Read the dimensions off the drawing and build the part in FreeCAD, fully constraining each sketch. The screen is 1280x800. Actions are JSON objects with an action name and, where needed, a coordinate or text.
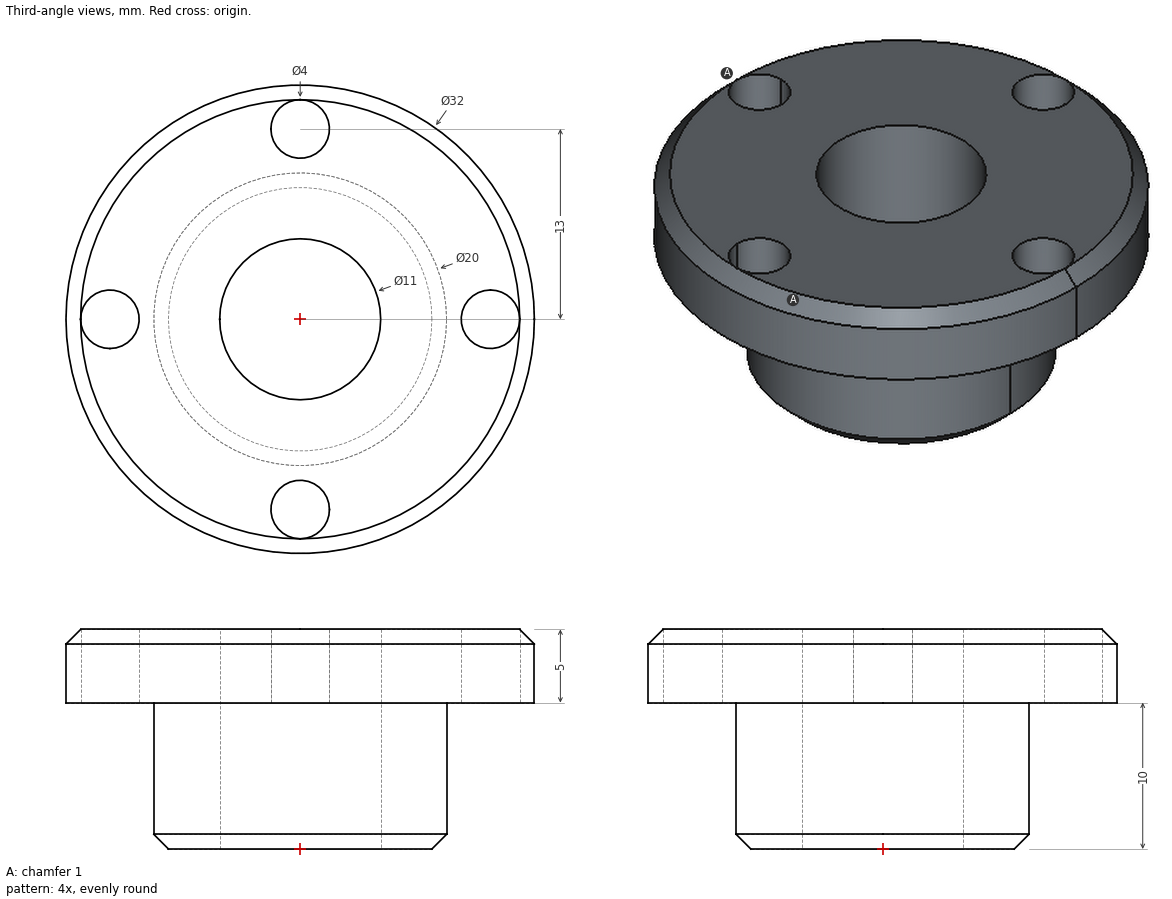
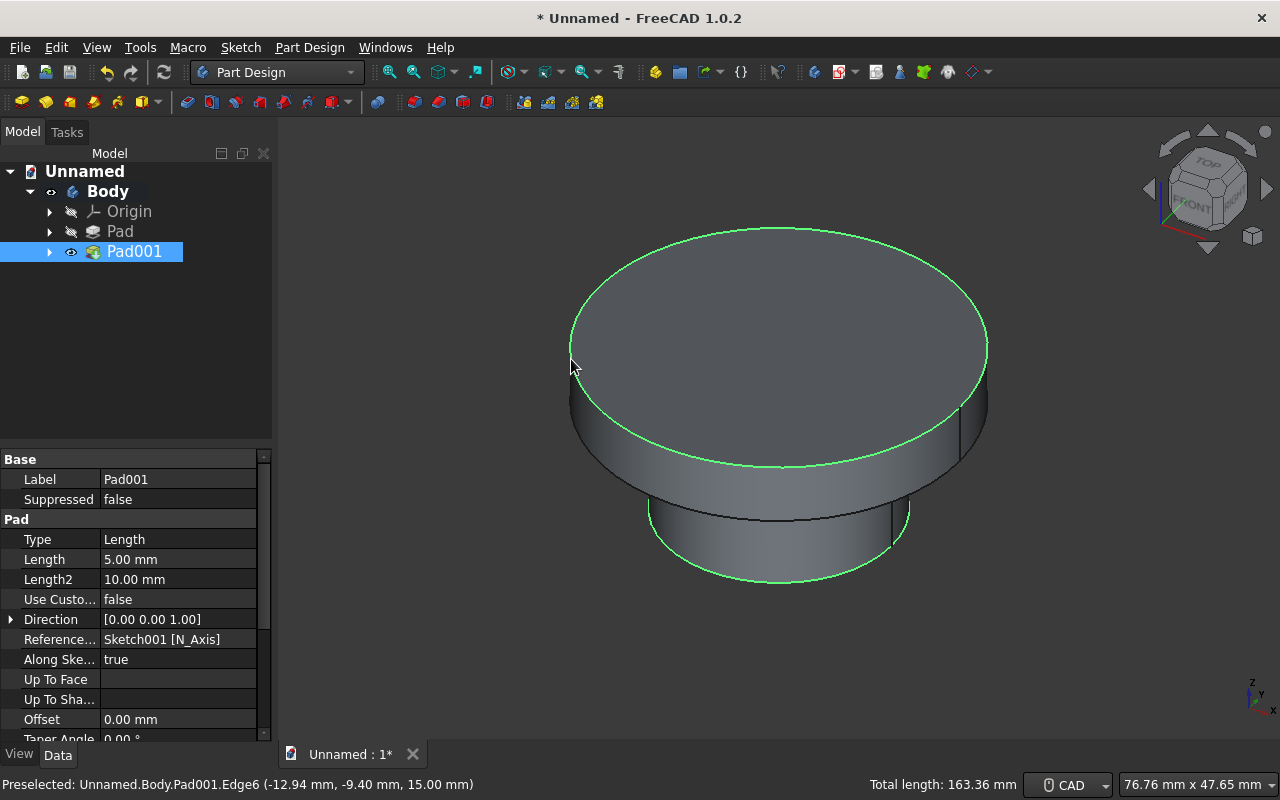
{"action": "left_click", "coordinate": [440, 102]}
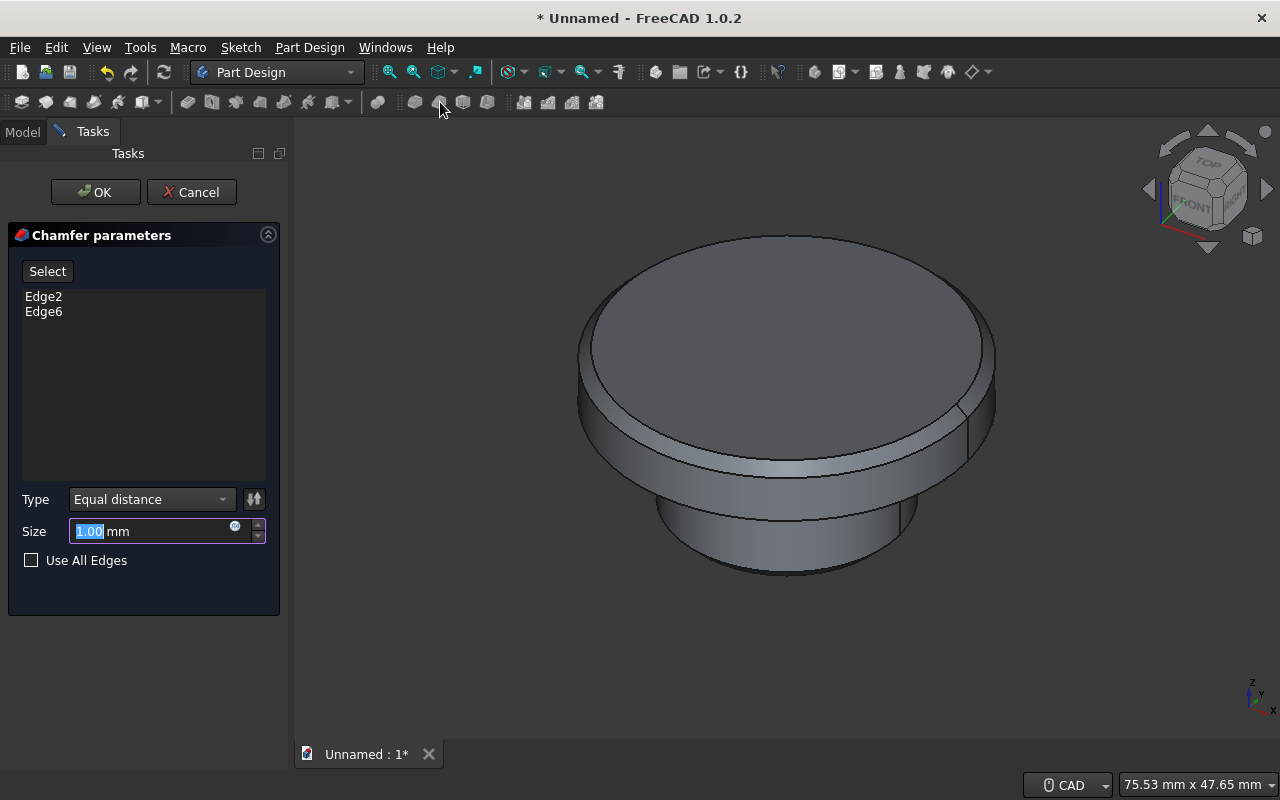
{"action": "type", "text": "1"}
{"action": "key", "text": "Tab"}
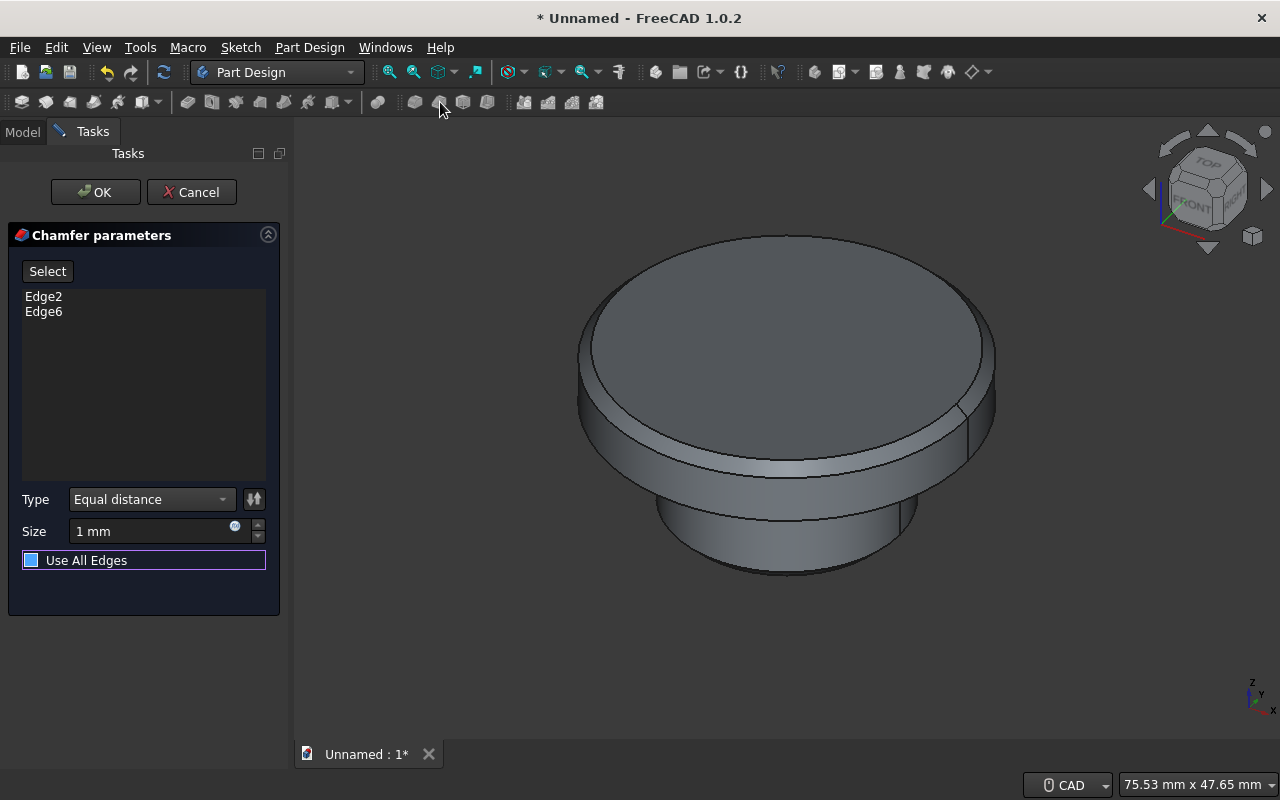
{"action": "left_click", "coordinate": [96, 192]}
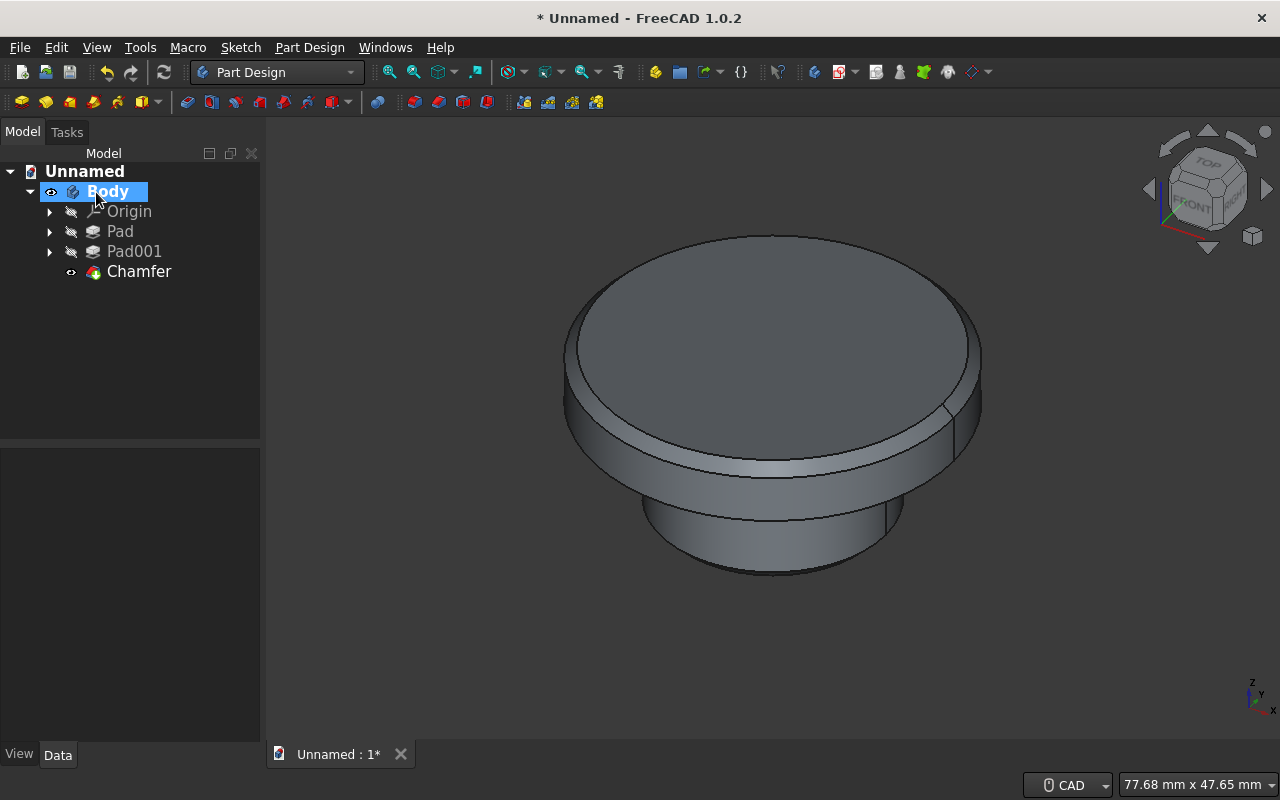
{"action": "key", "text": "5"}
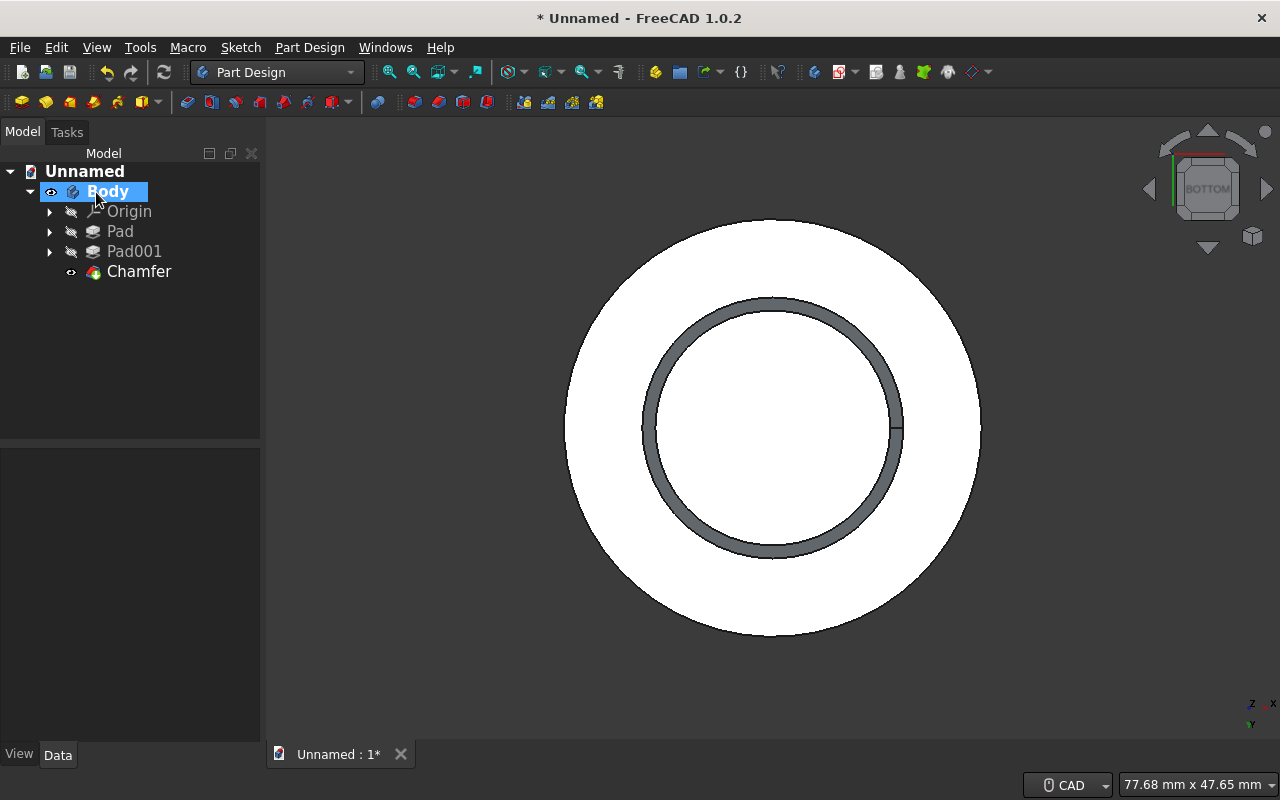
{"action": "left_click", "coordinate": [653, 546]}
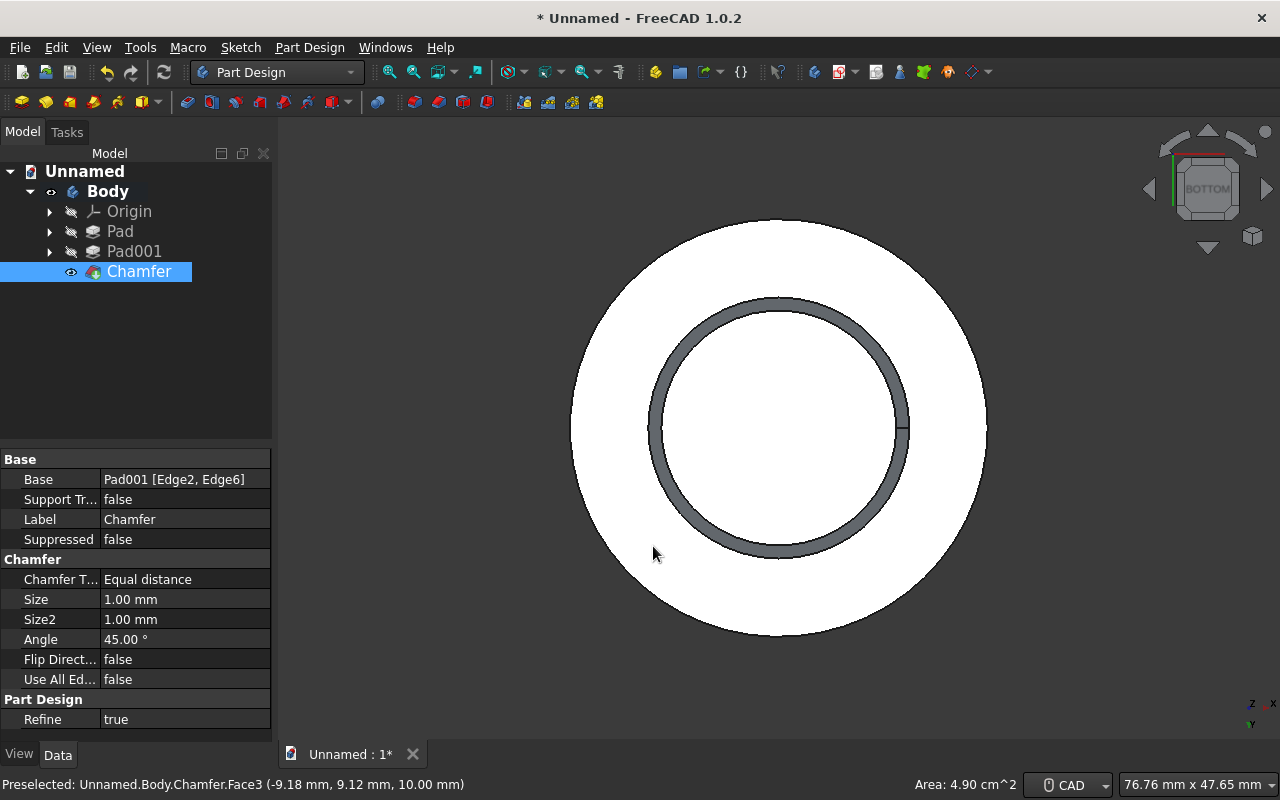
{"action": "left_click", "coordinate": [840, 72]}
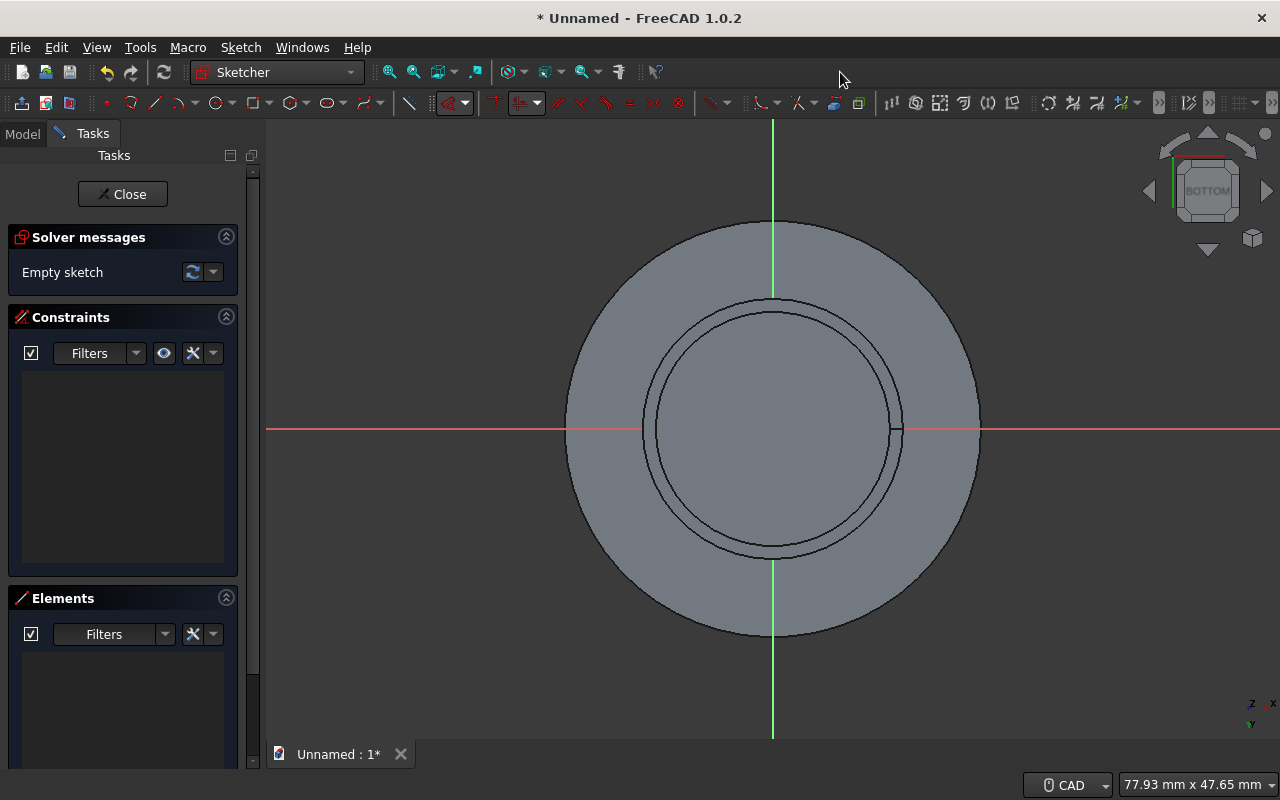
{"action": "left_click", "coordinate": [70, 104]}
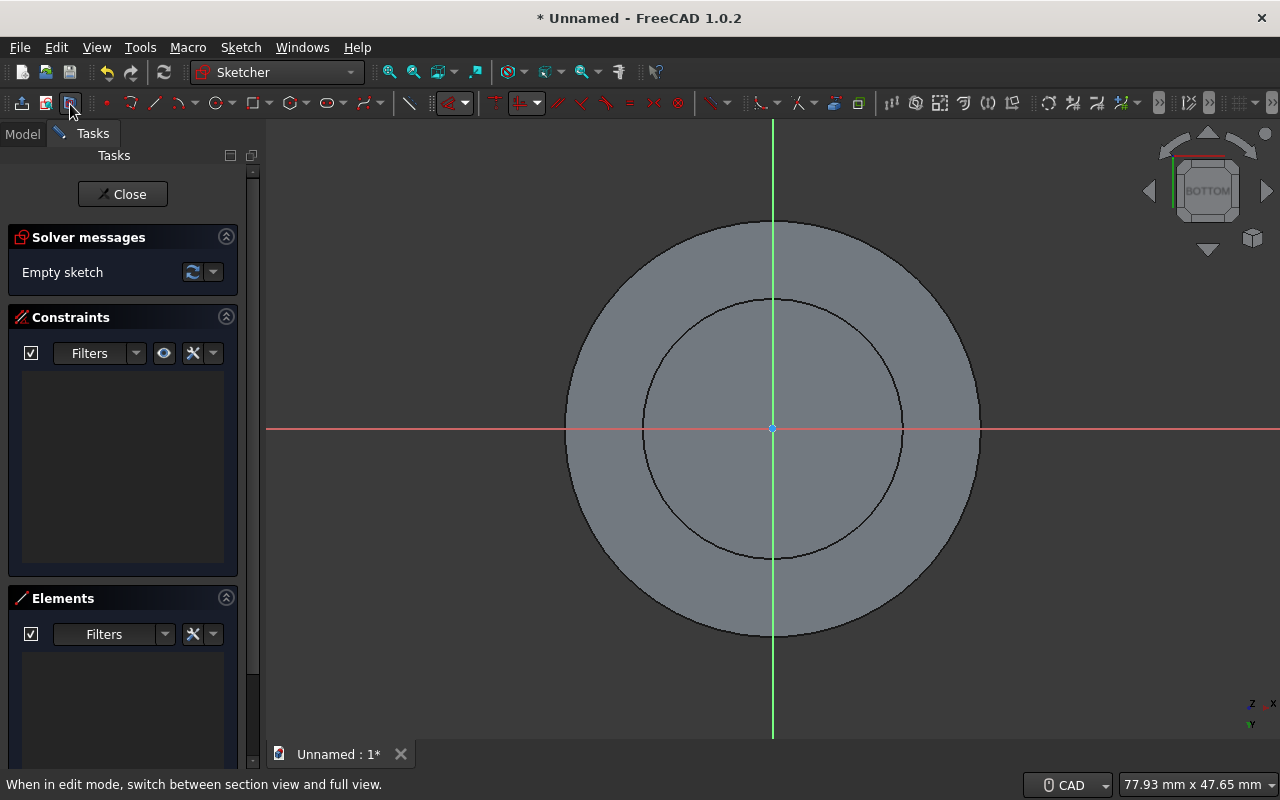
{"action": "scroll", "coordinate": [784, 625], "scroll_direction": "up", "scroll_amount": 10}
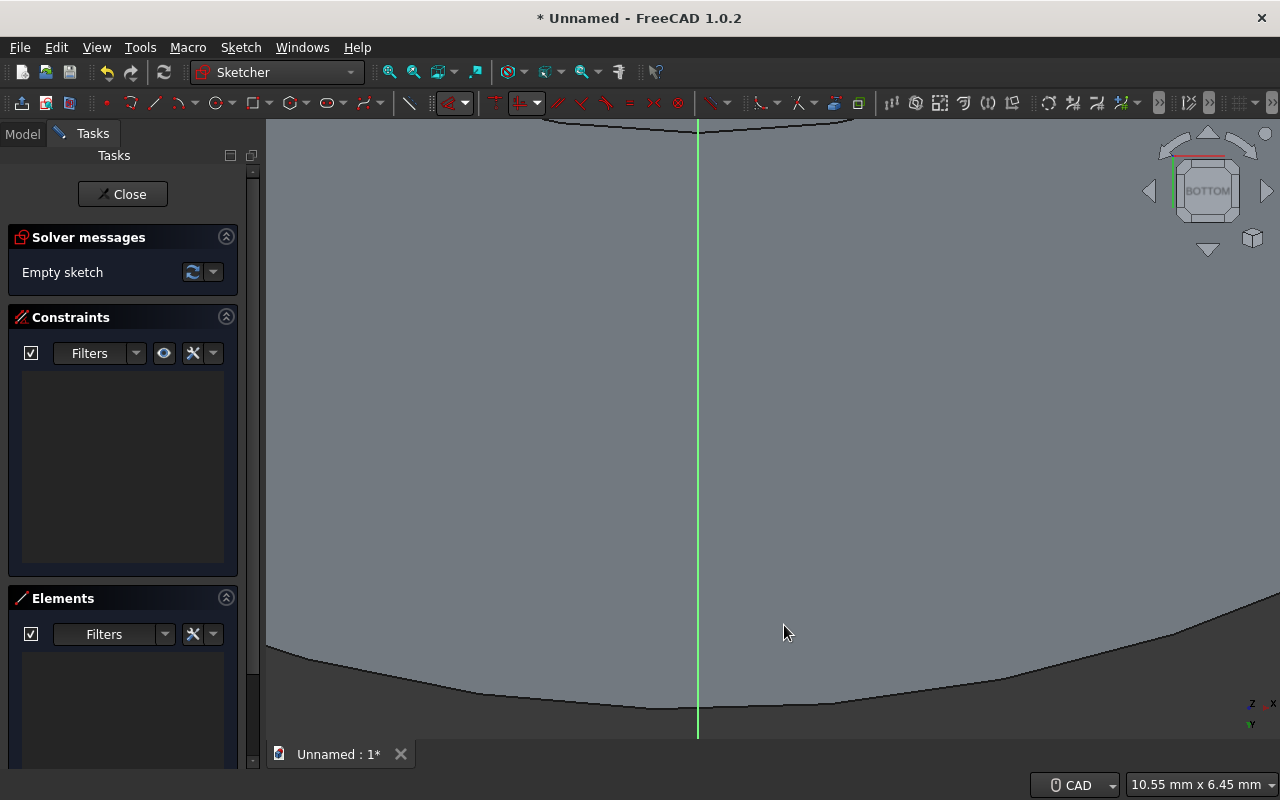
{"action": "key", "text": "g c"}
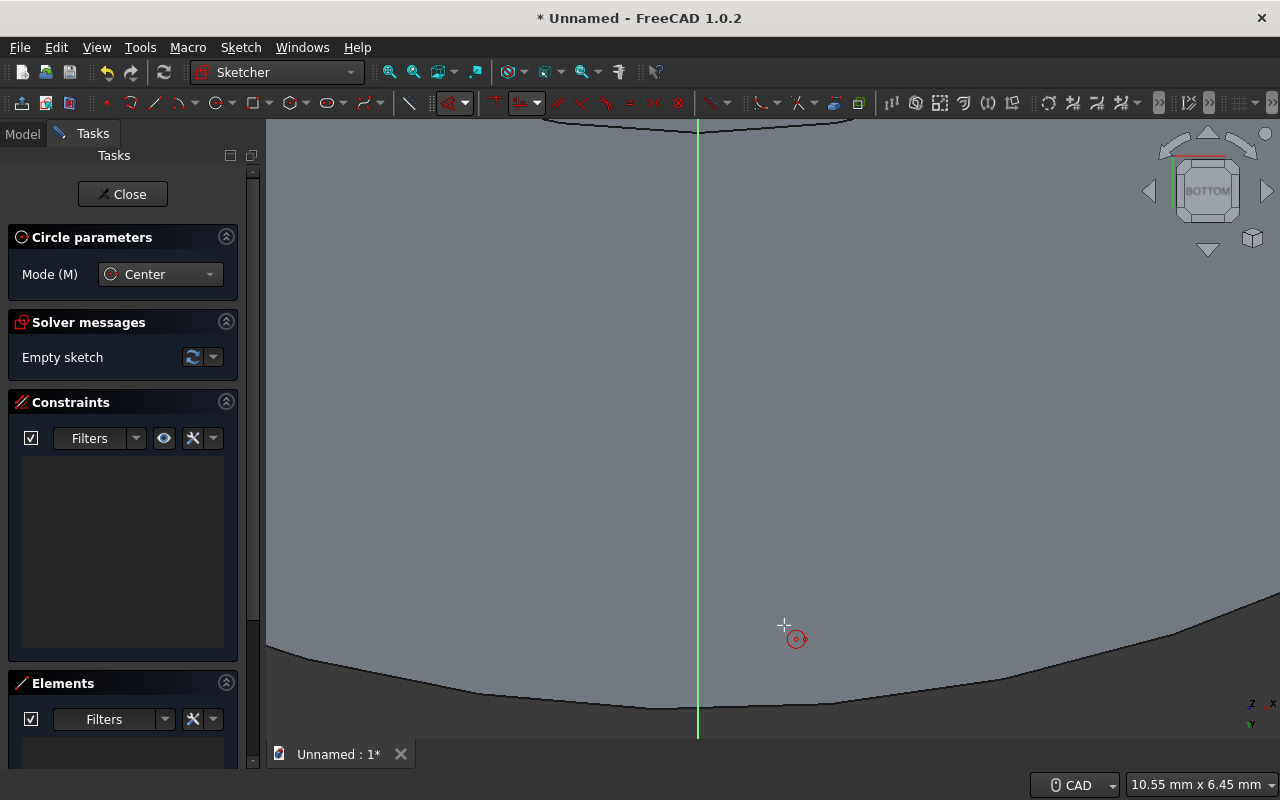
{"action": "left_click", "coordinate": [698, 421]}
{"action": "left_click", "coordinate": [834, 285]}
{"action": "key", "text": "Escape"}